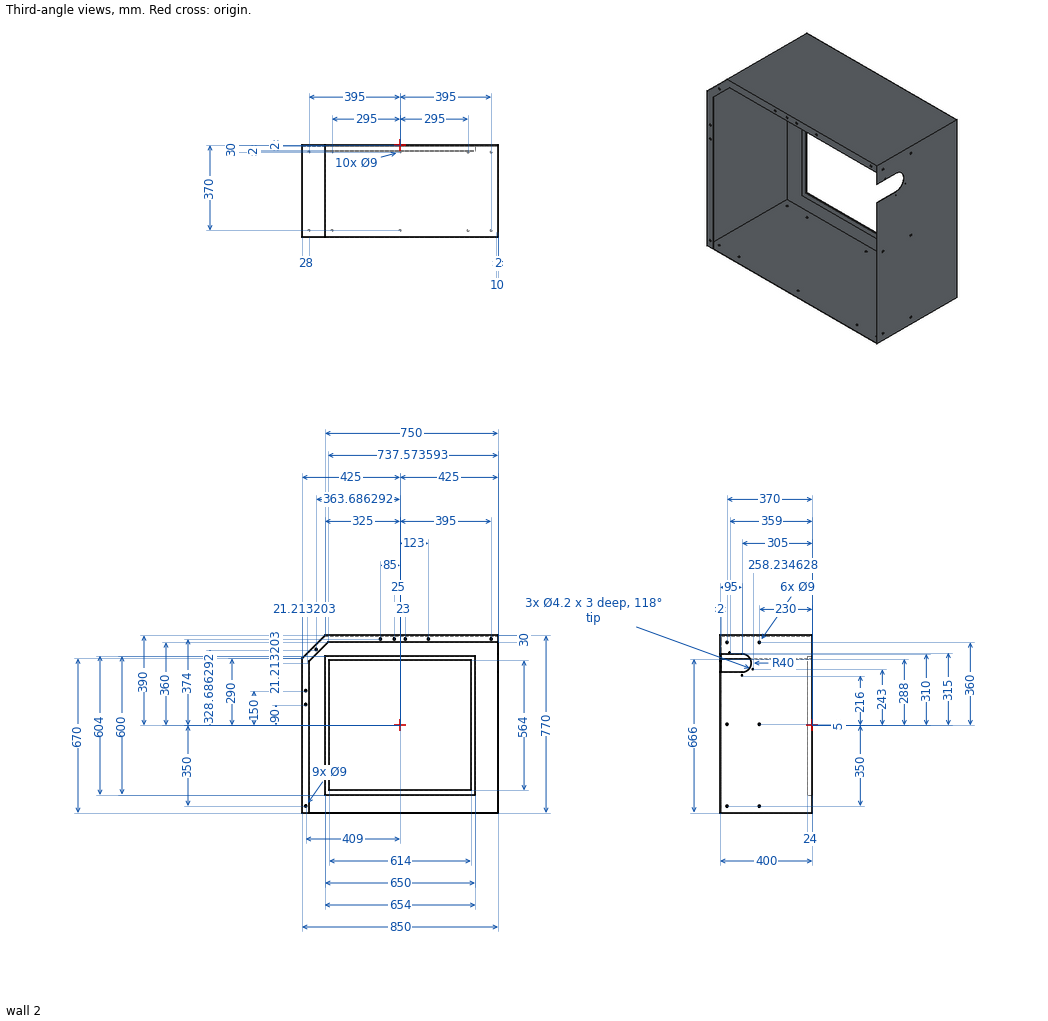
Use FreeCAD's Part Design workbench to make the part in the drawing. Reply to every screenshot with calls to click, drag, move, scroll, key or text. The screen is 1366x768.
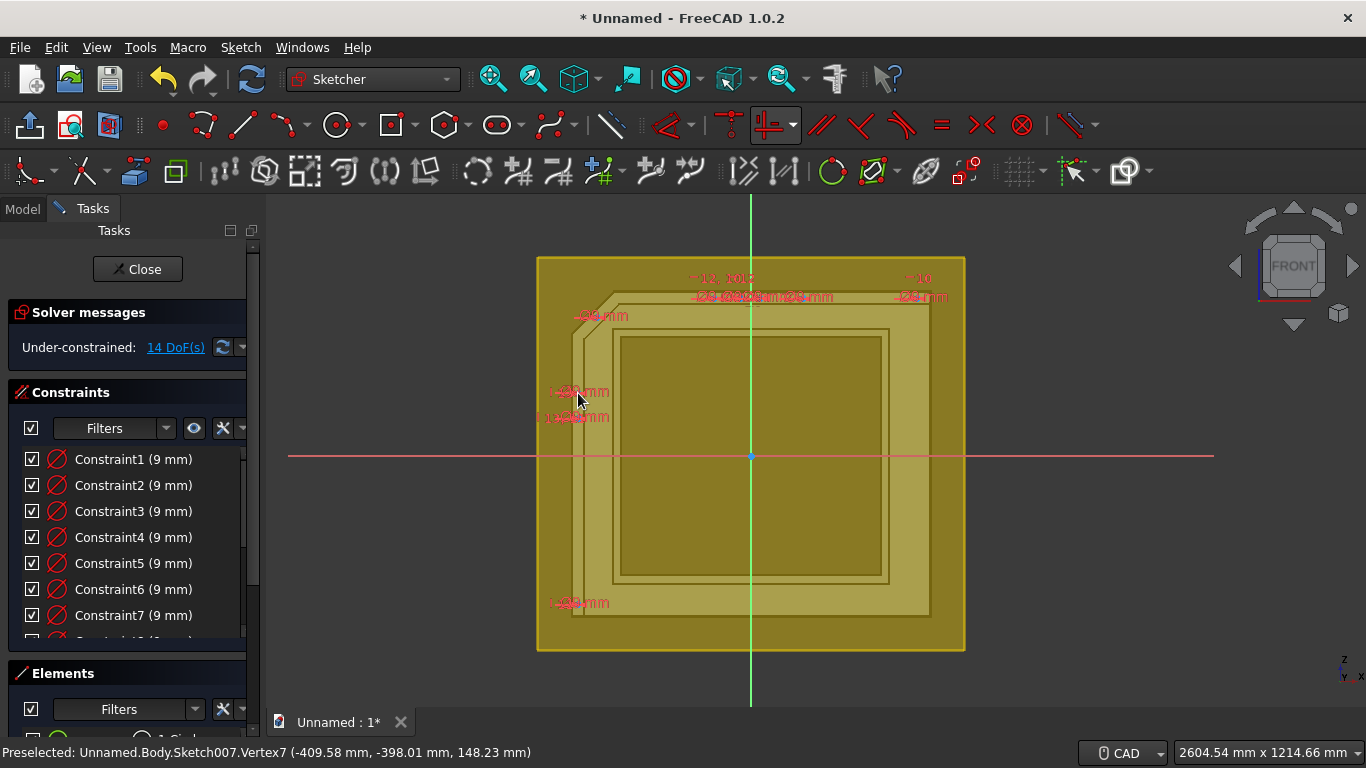
click(740, 299)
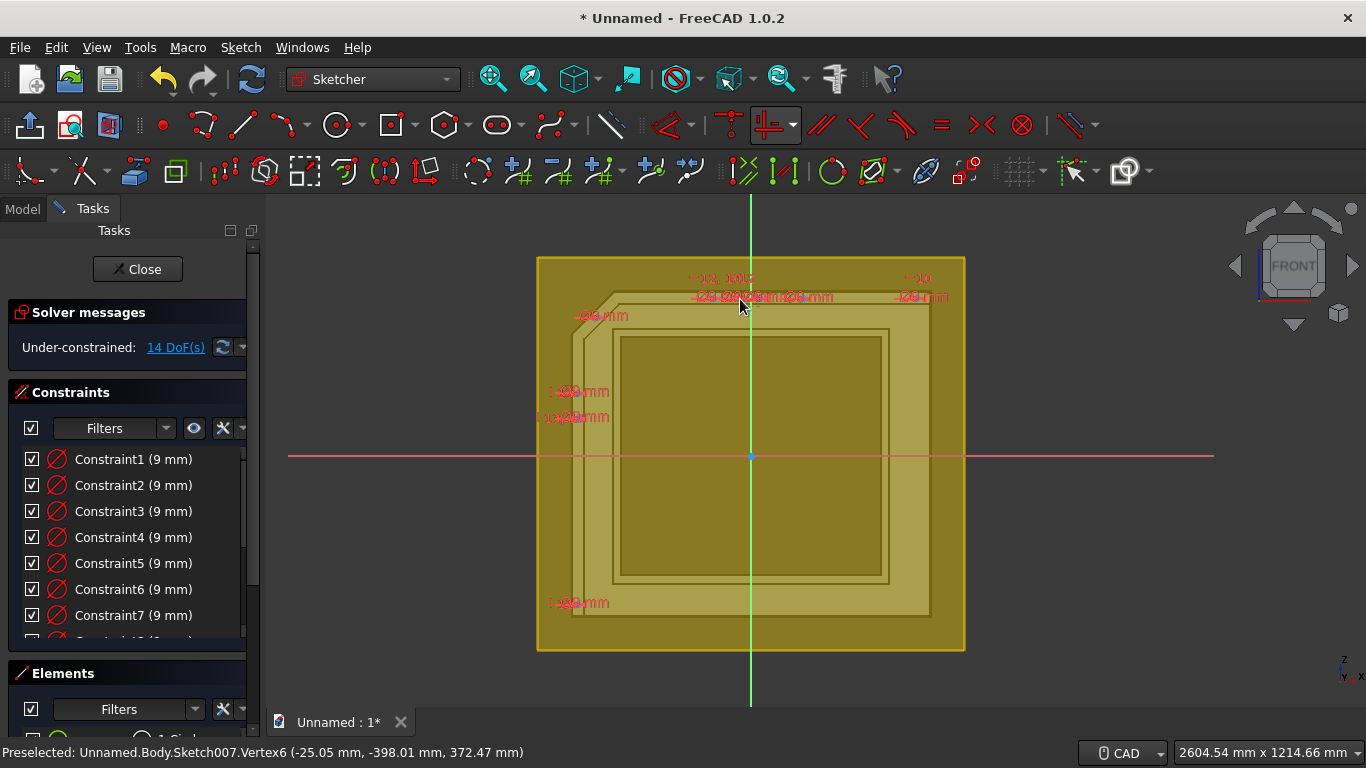
click(761, 299)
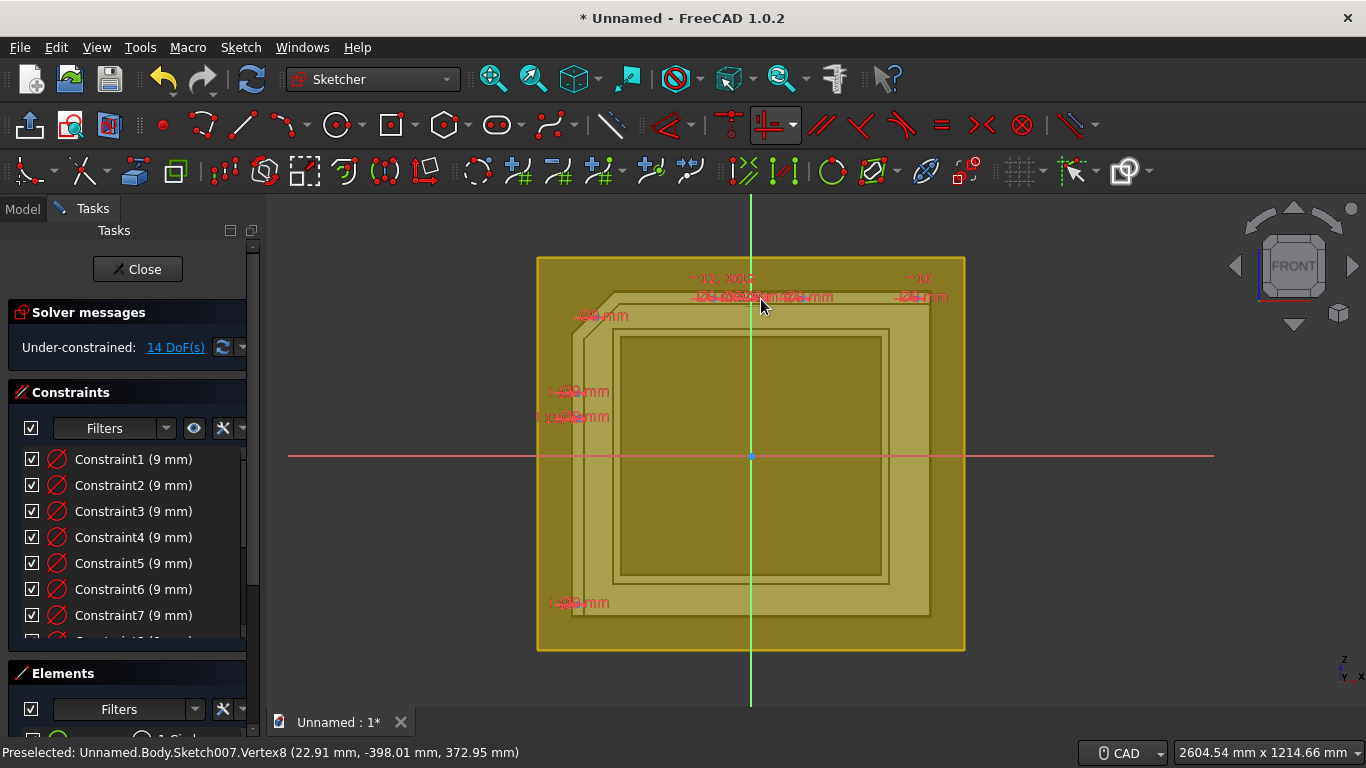
click(796, 126)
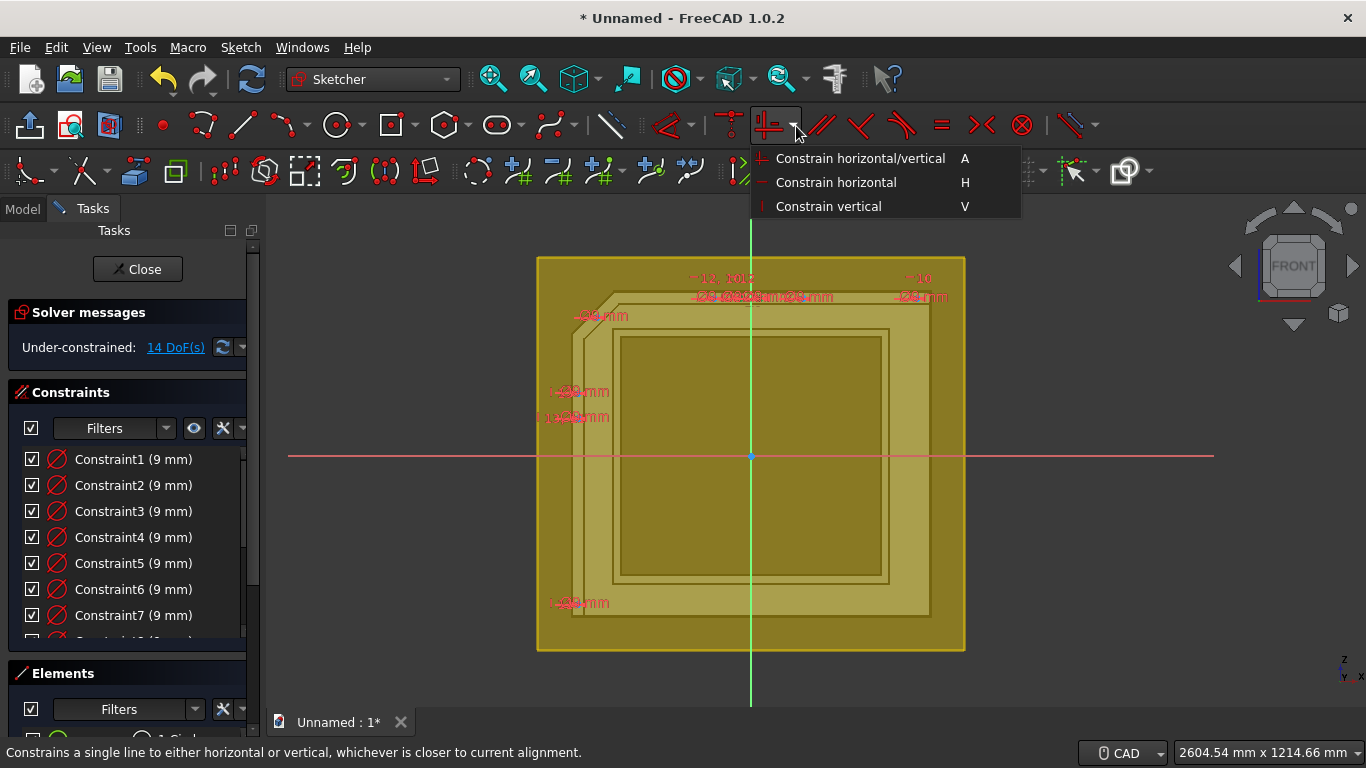
click(886, 182)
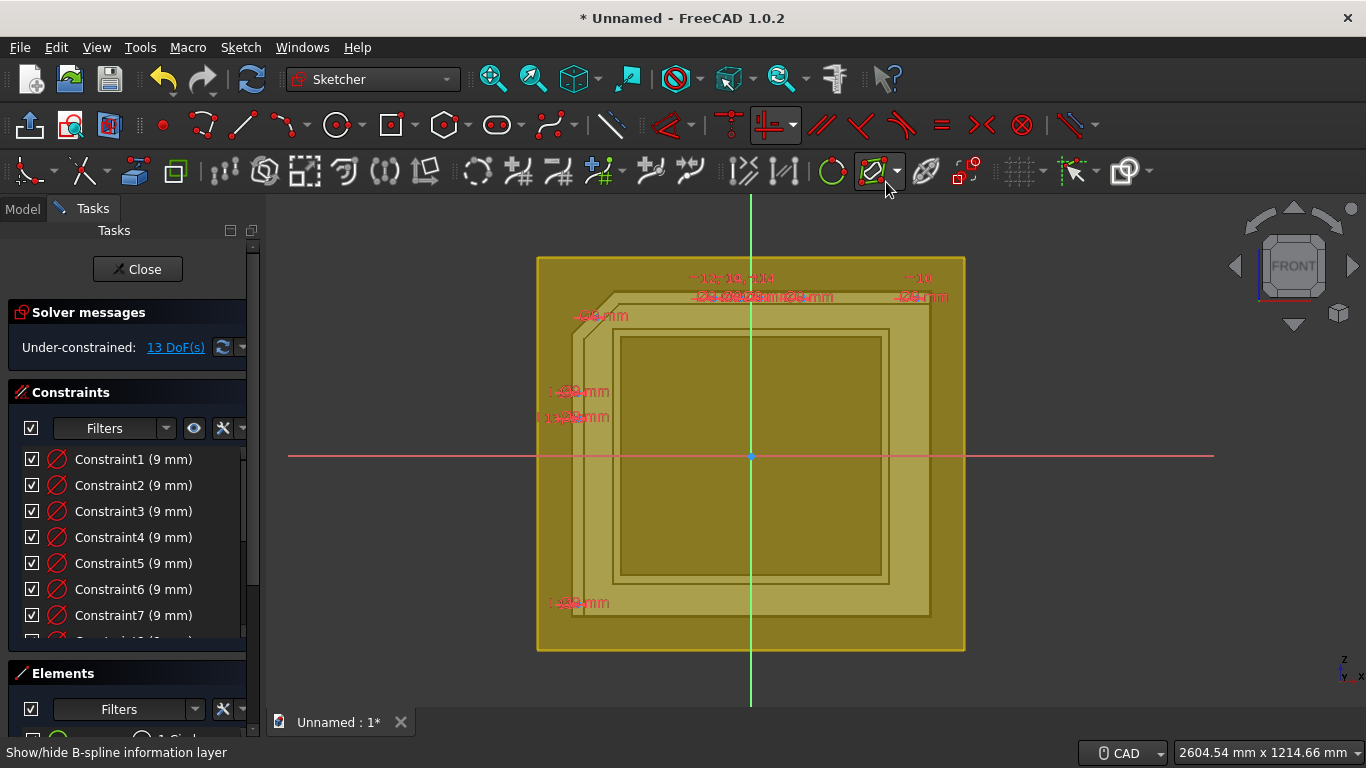
click(761, 299)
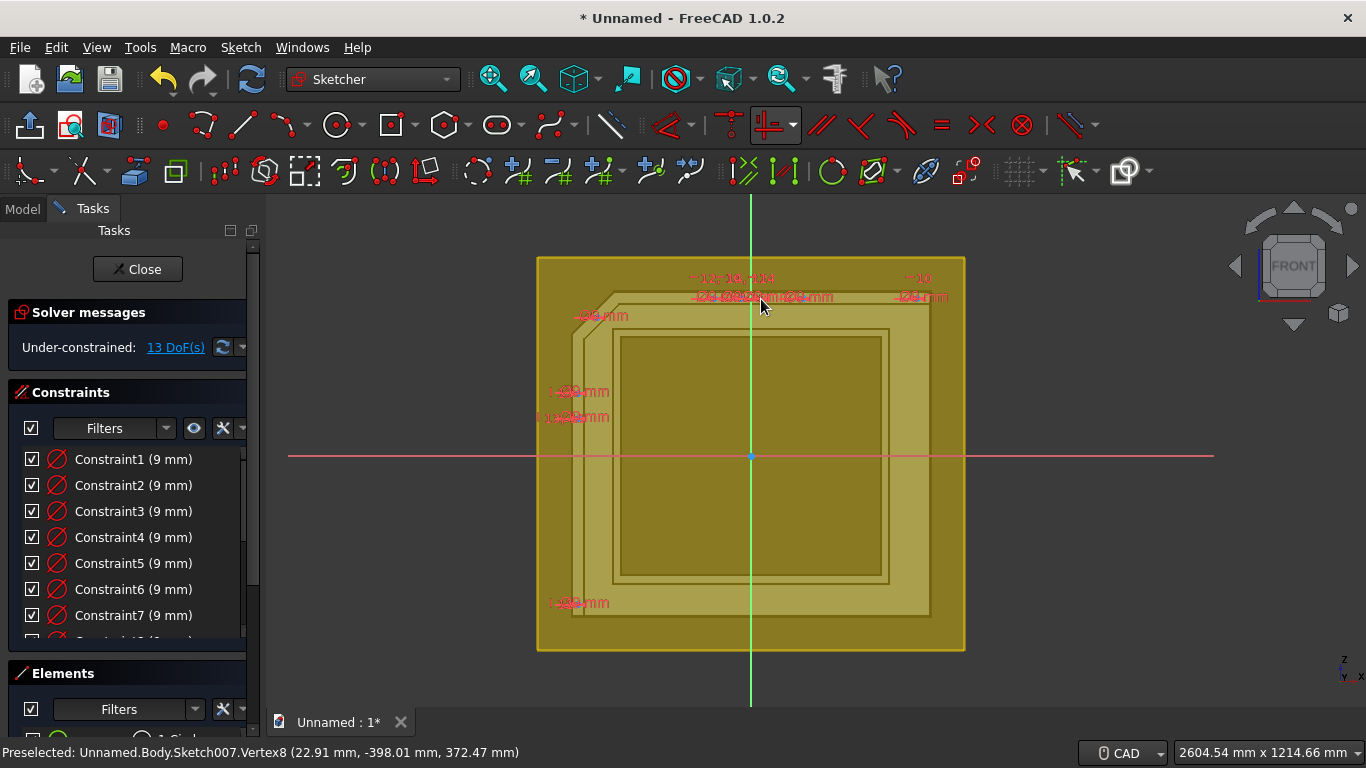
click(803, 299)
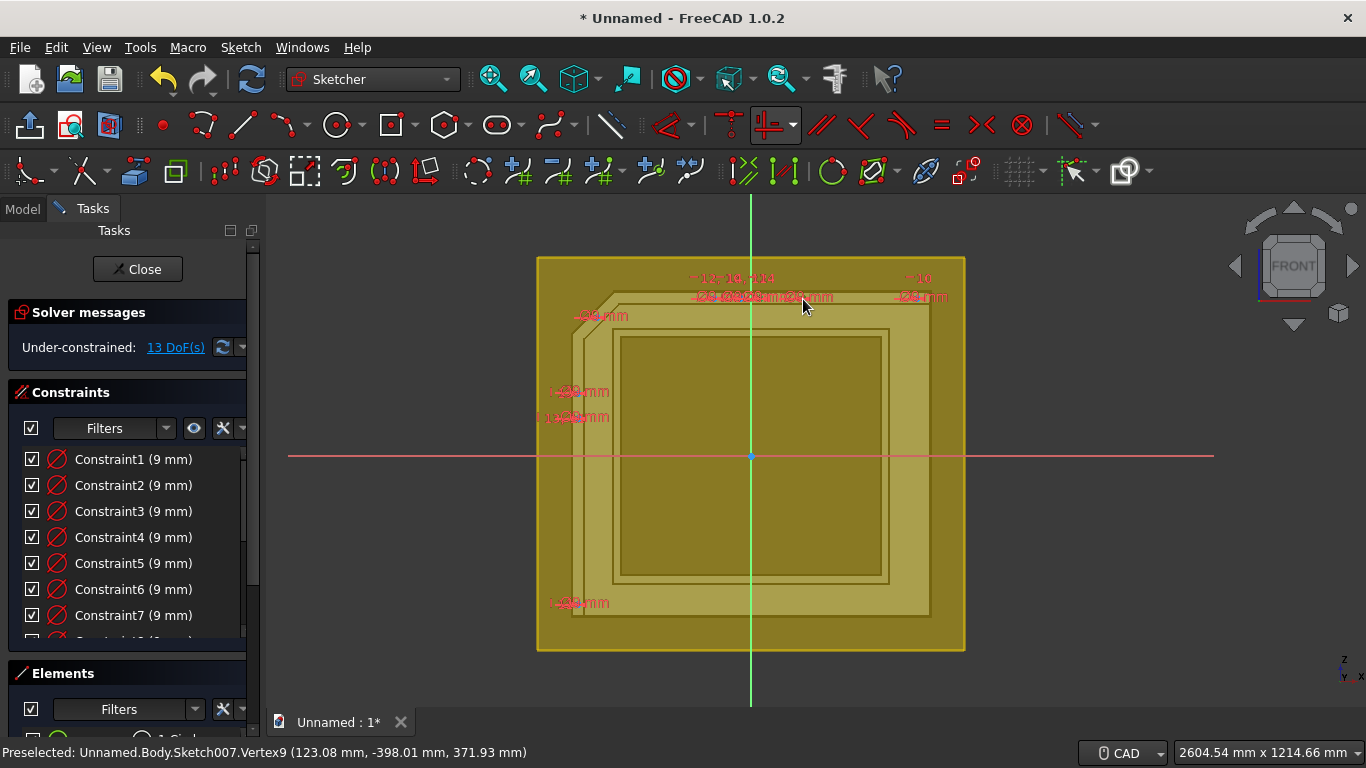
click(796, 126)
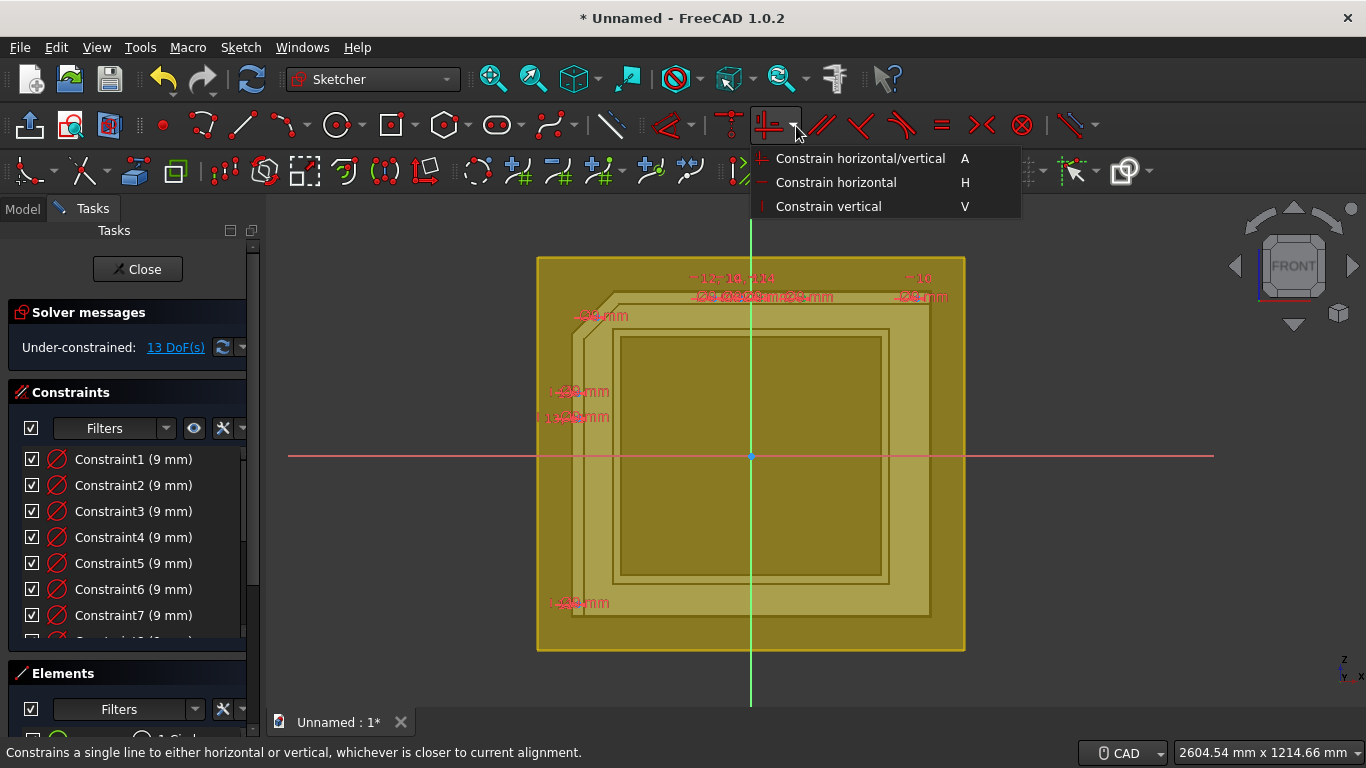
click(886, 182)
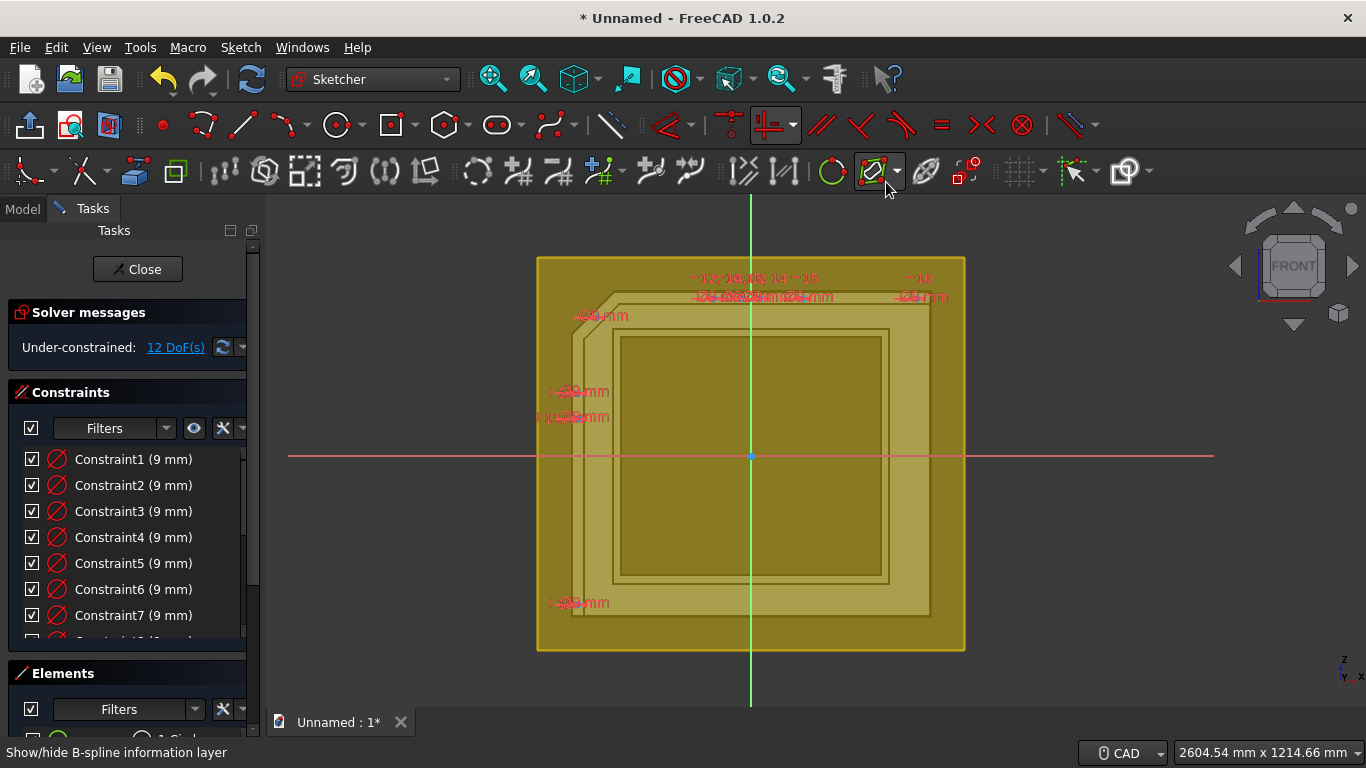
click(666, 126)